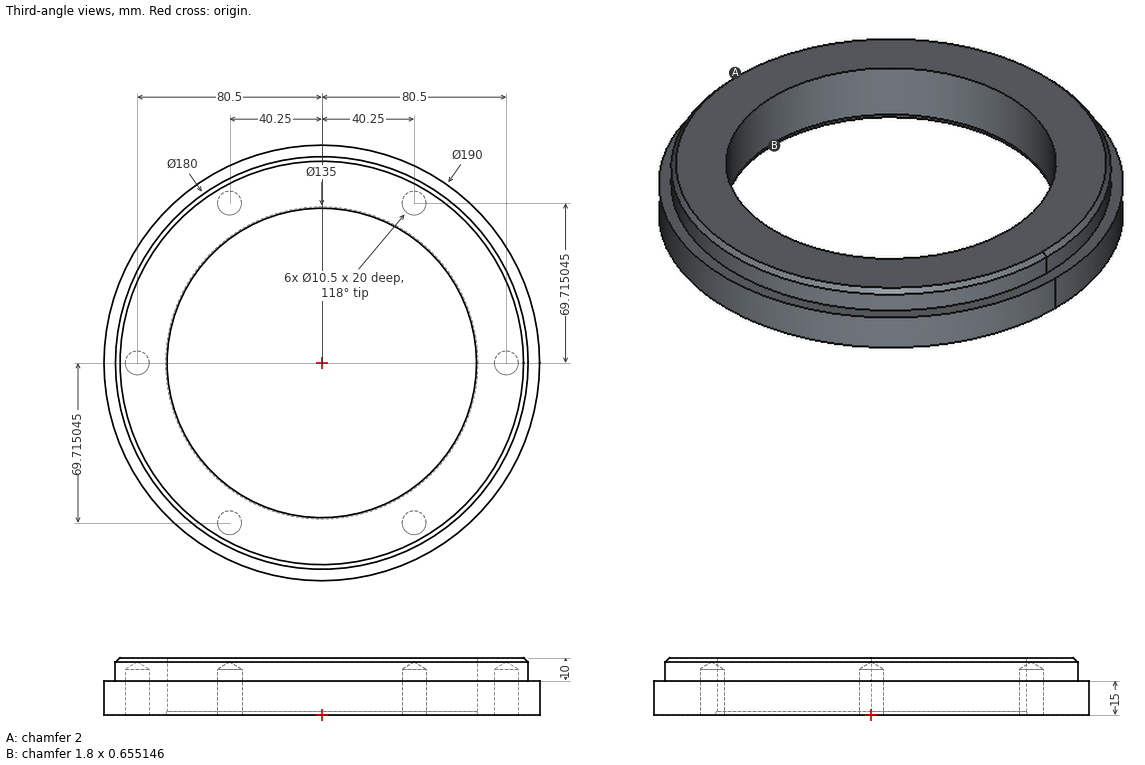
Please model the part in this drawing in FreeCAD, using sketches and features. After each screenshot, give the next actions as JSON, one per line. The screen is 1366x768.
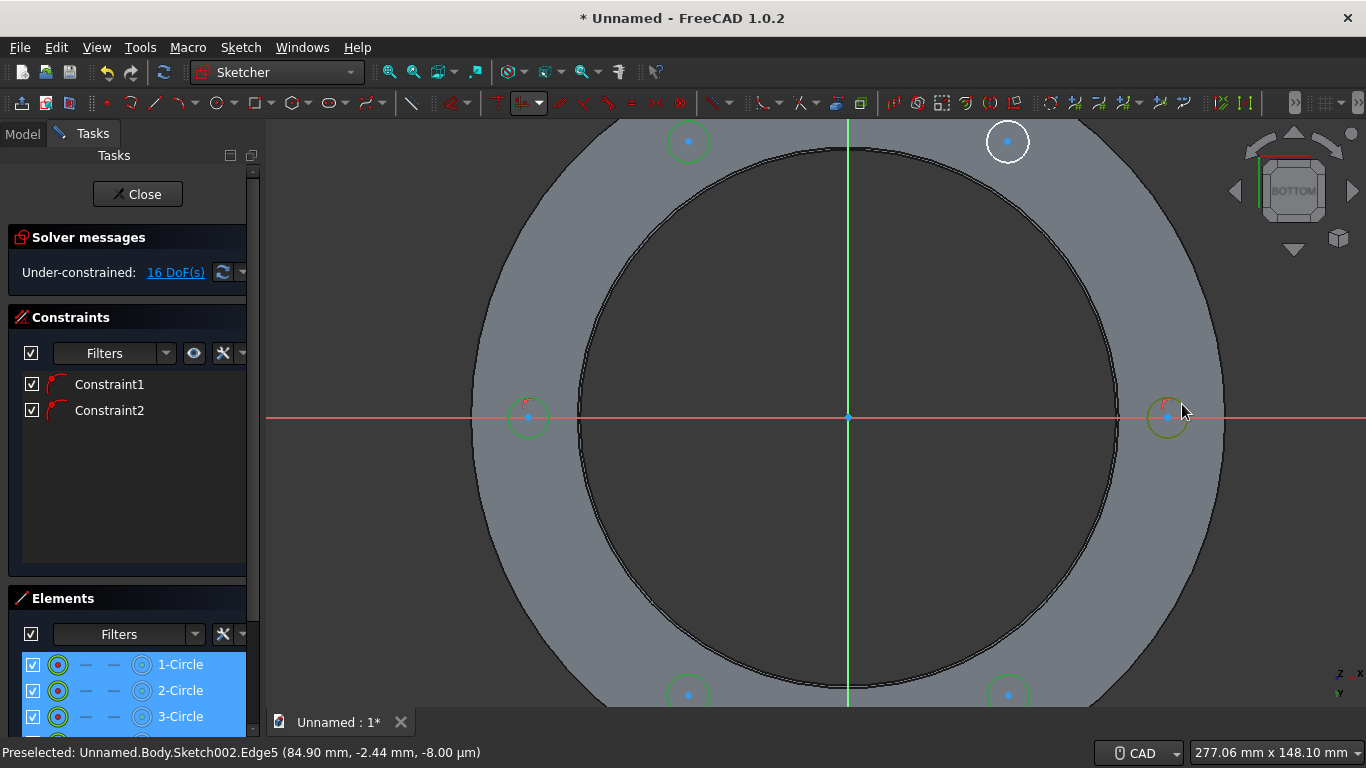
{"action": "left_click", "coordinate": [993, 157]}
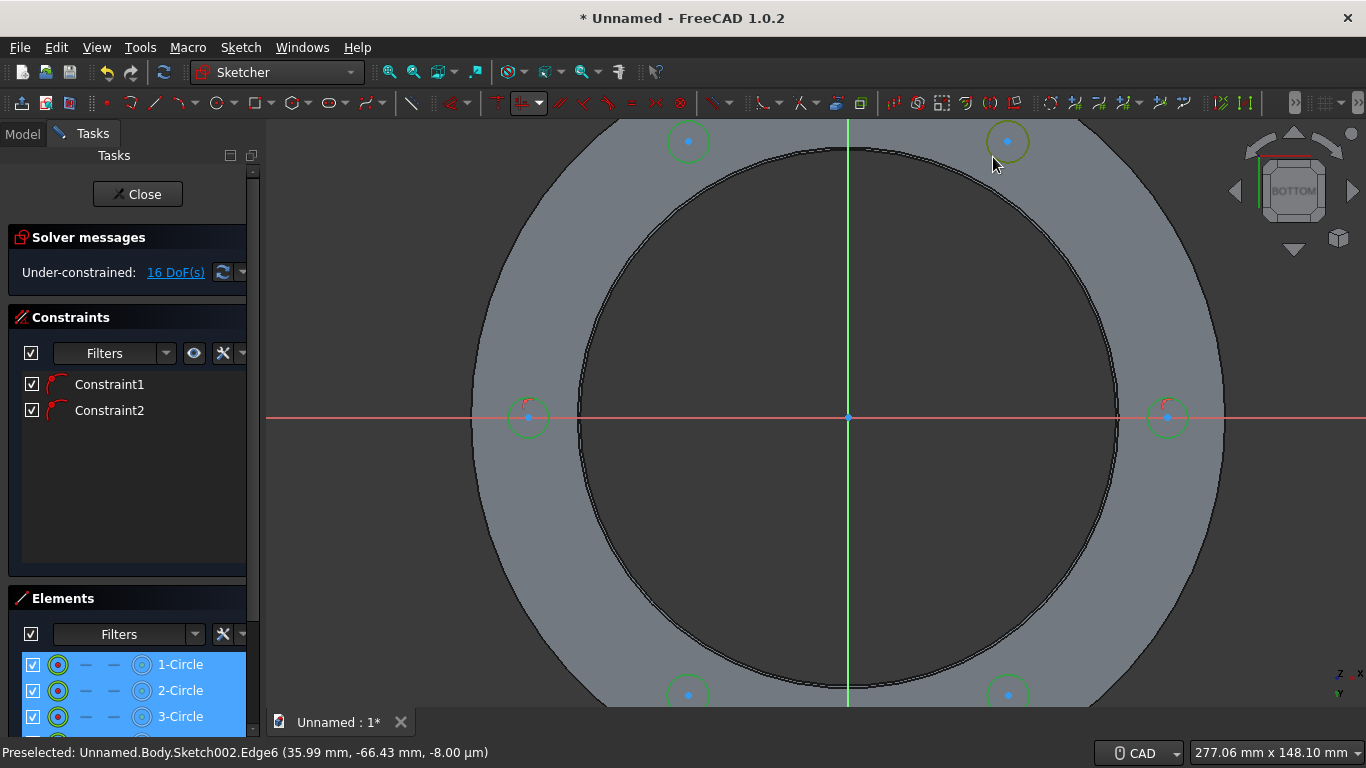
{"action": "left_click", "coordinate": [632, 104]}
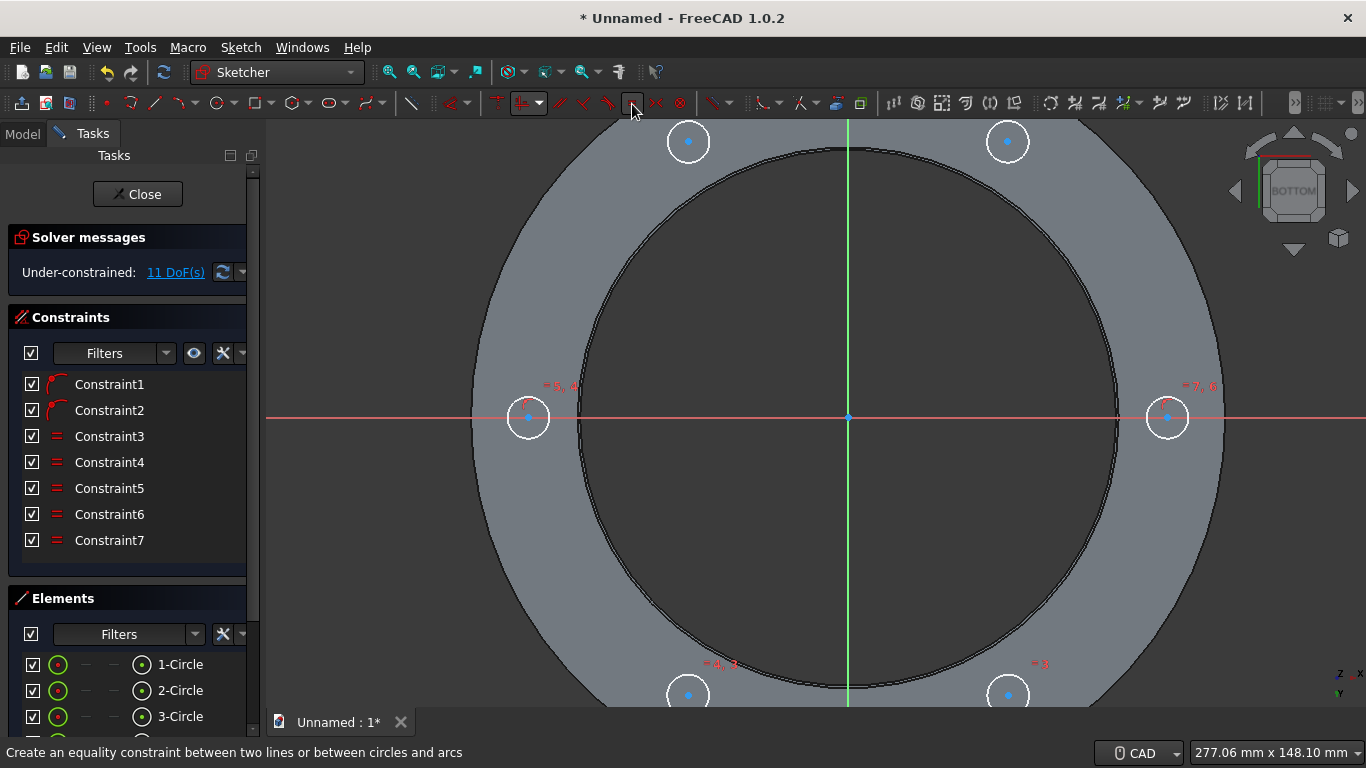
{"action": "scroll", "coordinate": [543, 403], "scroll_direction": "down", "scroll_amount": 2}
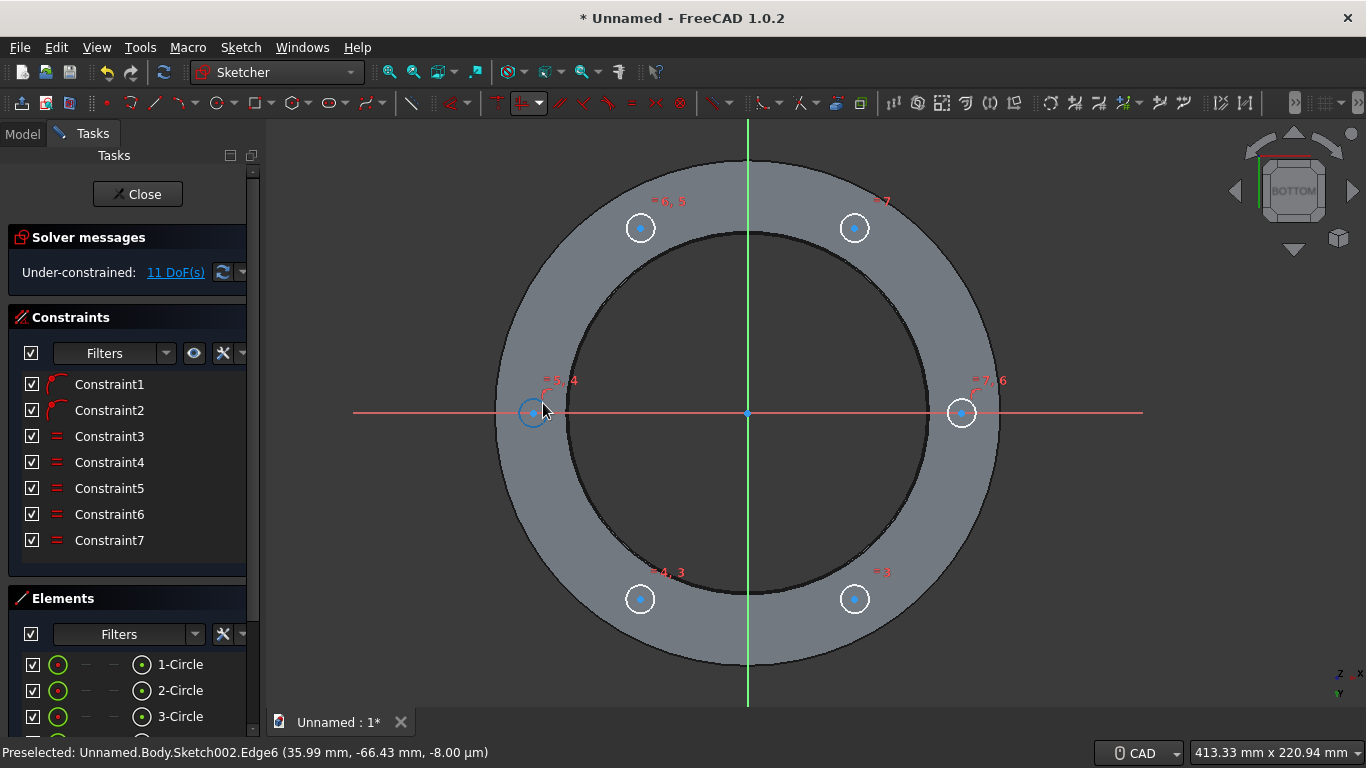
{"action": "left_click", "coordinate": [855, 599]}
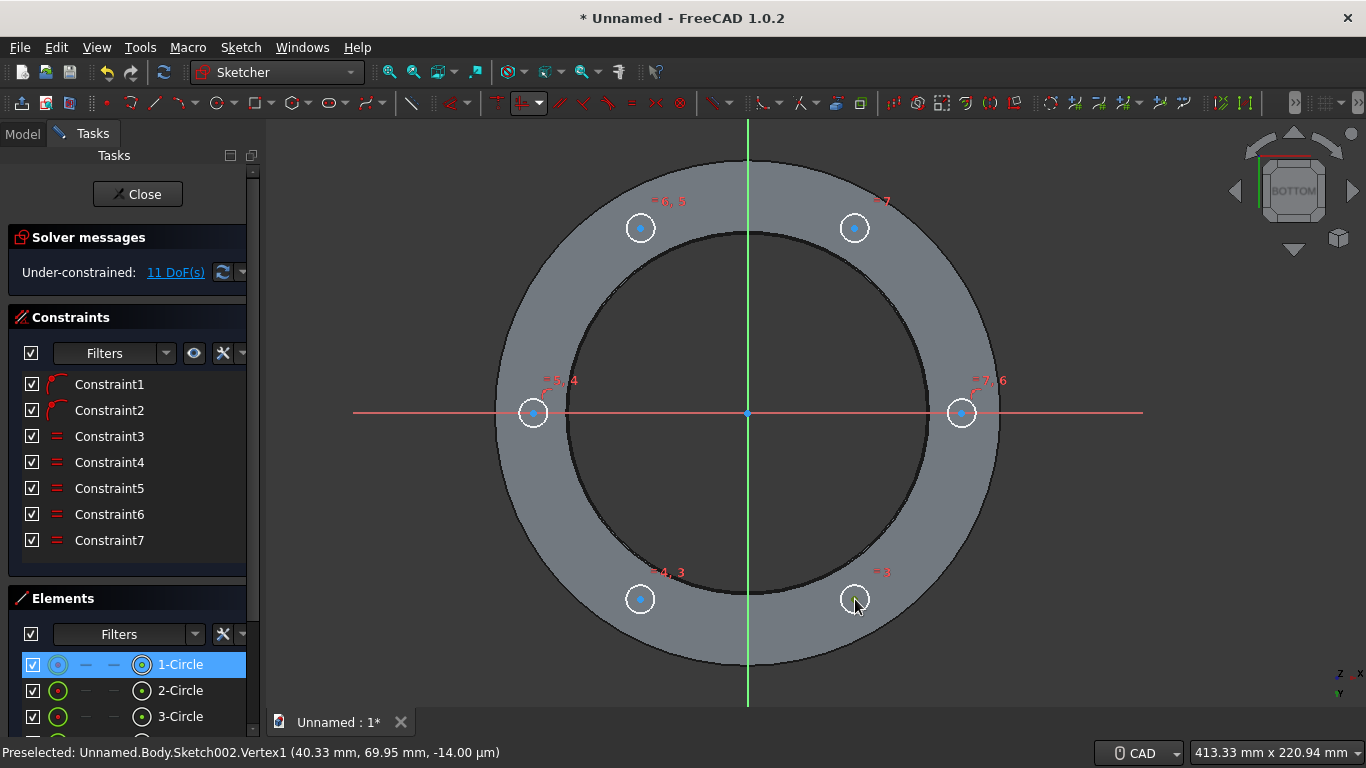
{"action": "left_click", "coordinate": [640, 599]}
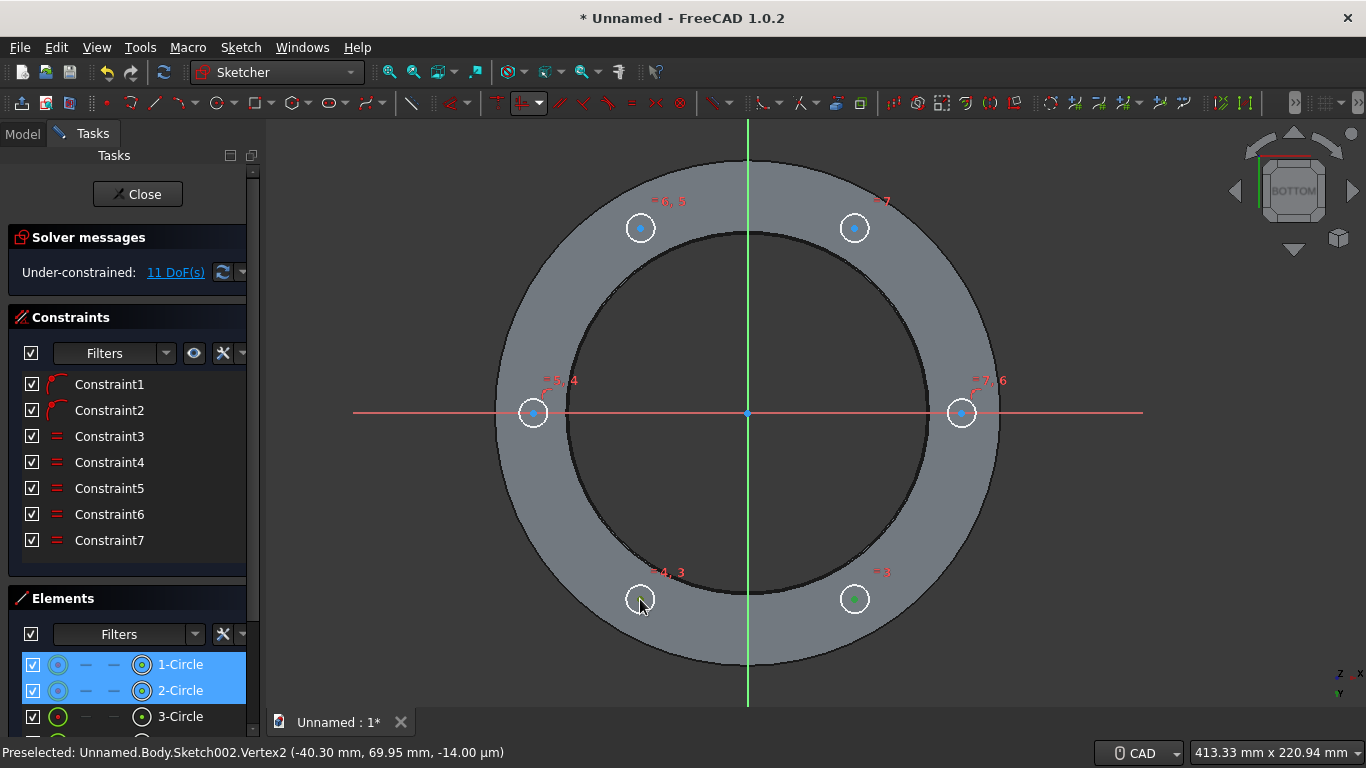
{"action": "left_click", "coordinate": [542, 104]}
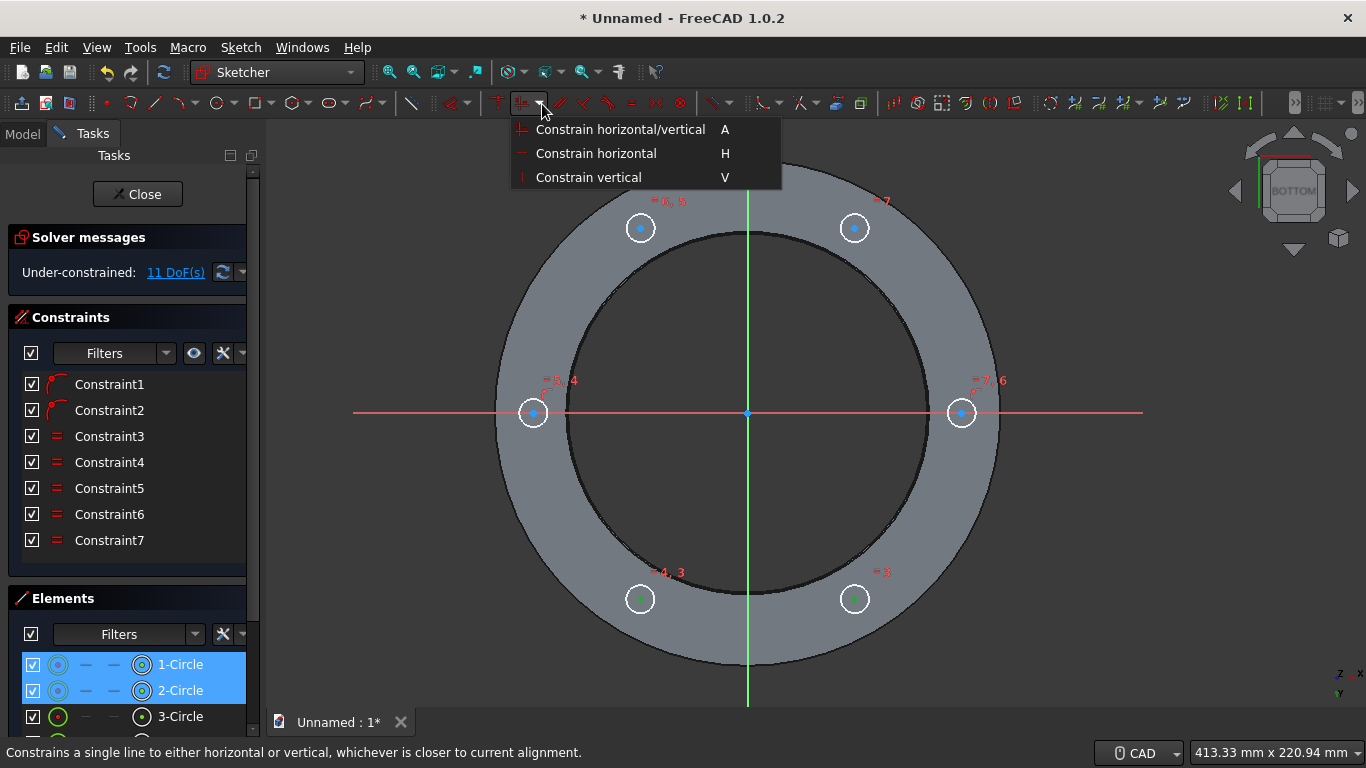
{"action": "left_click", "coordinate": [646, 153]}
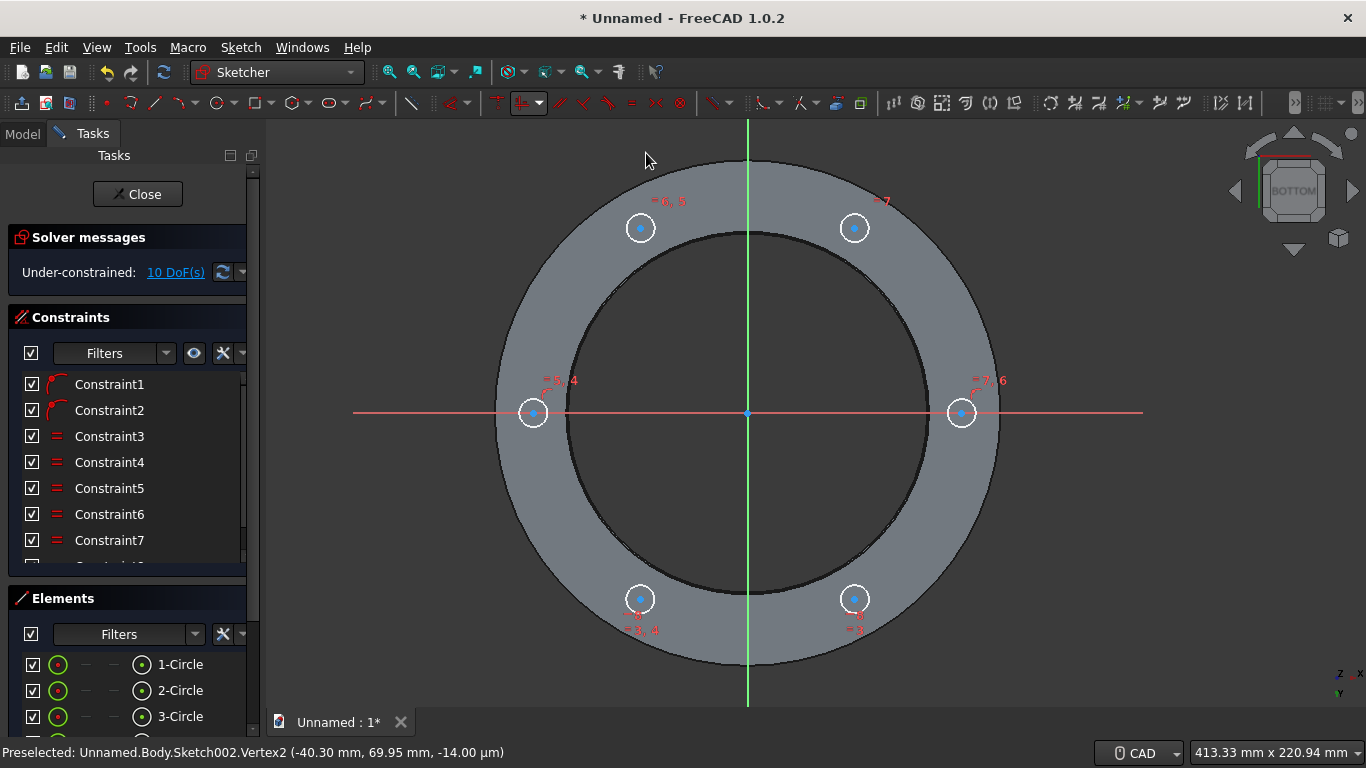
{"action": "left_click", "coordinate": [640, 599]}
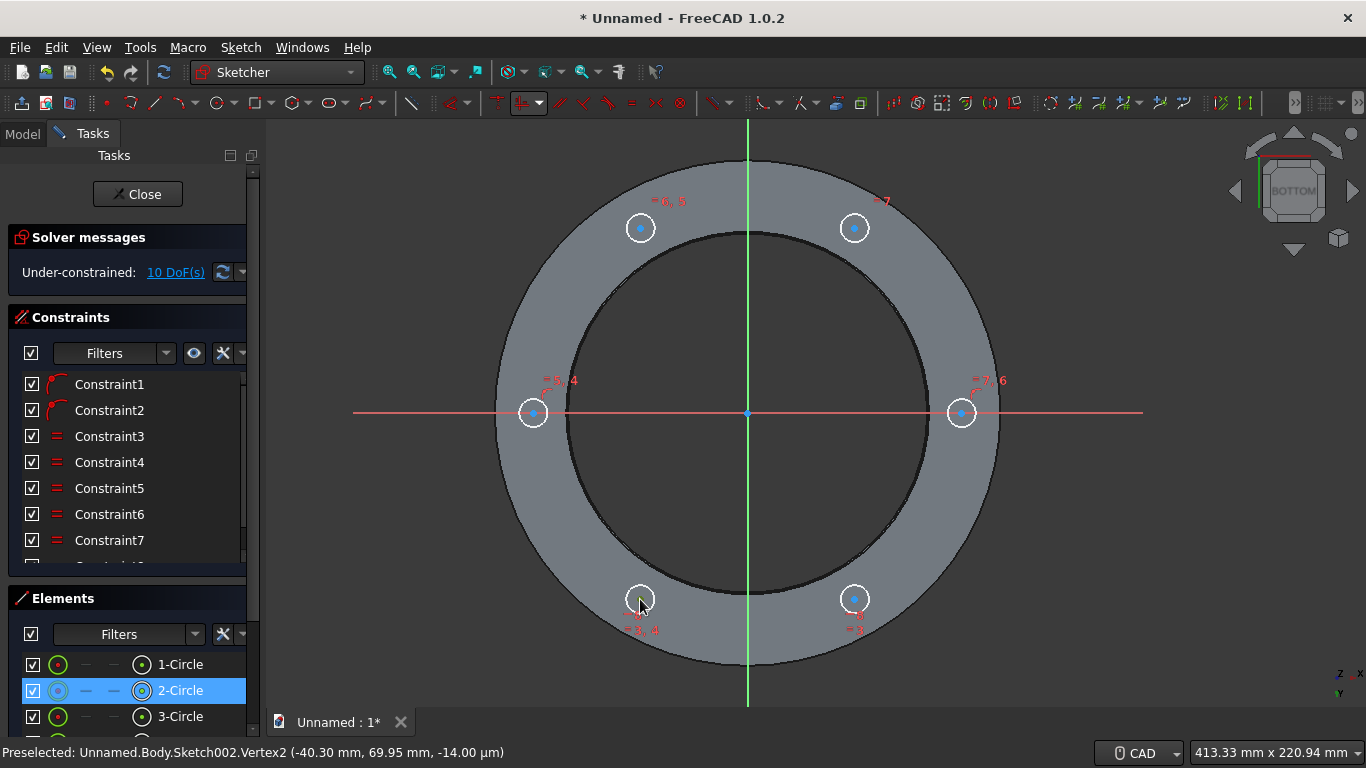
{"action": "left_click", "coordinate": [641, 228]}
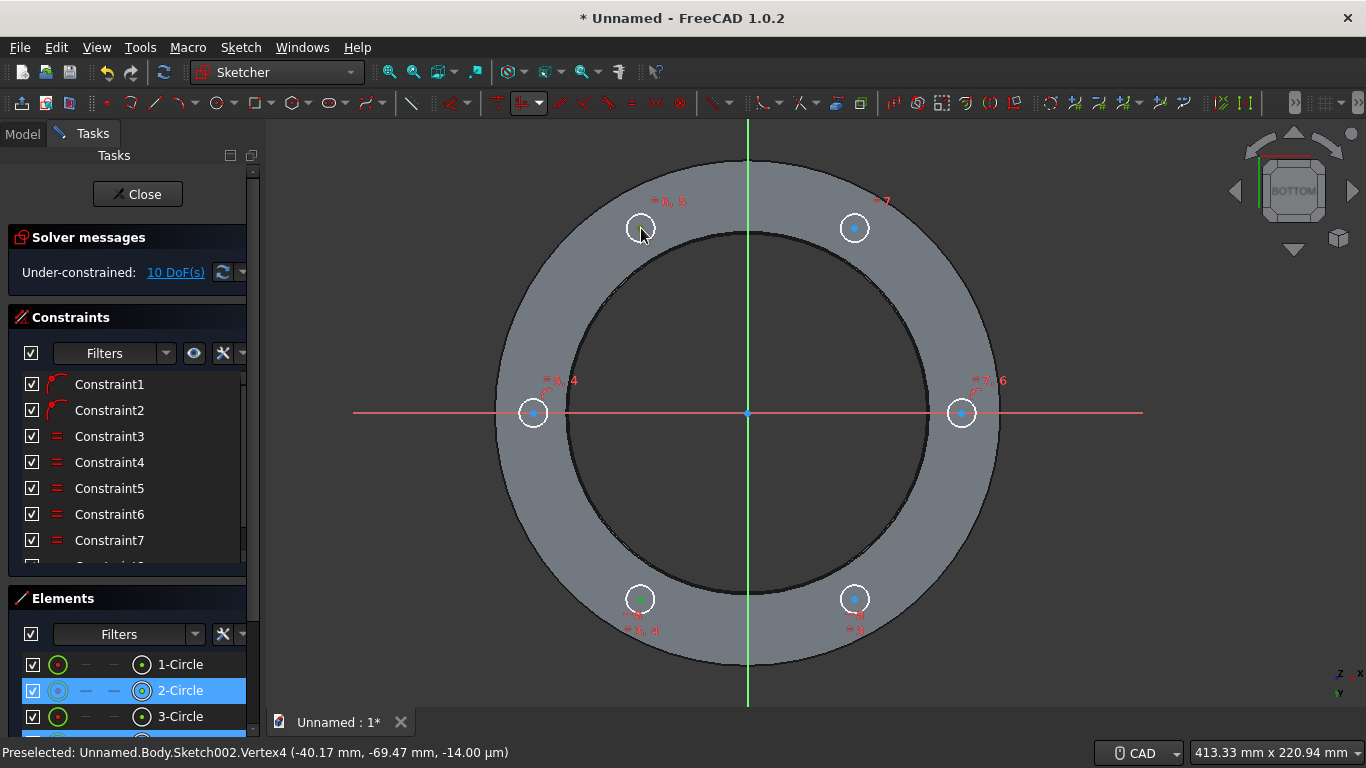
{"action": "left_click", "coordinate": [542, 104]}